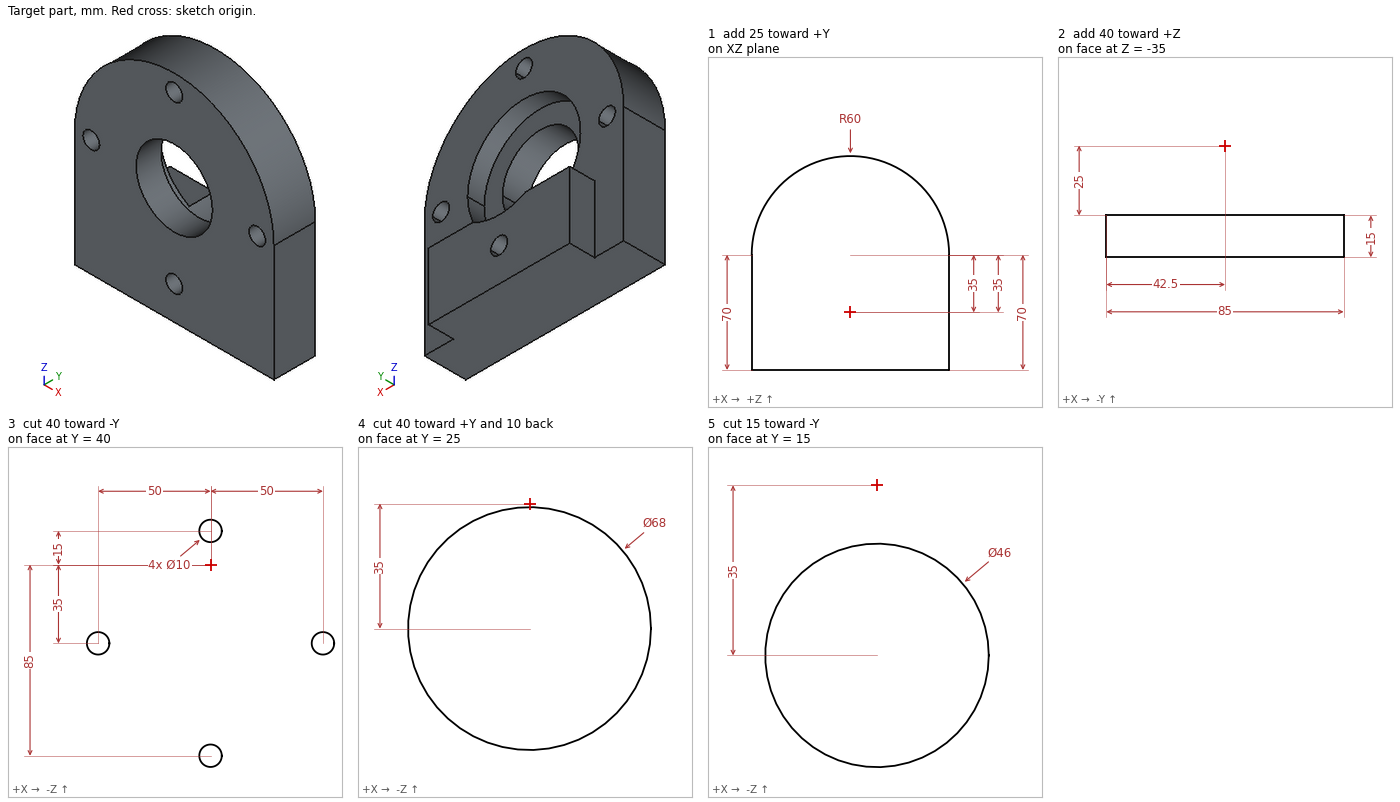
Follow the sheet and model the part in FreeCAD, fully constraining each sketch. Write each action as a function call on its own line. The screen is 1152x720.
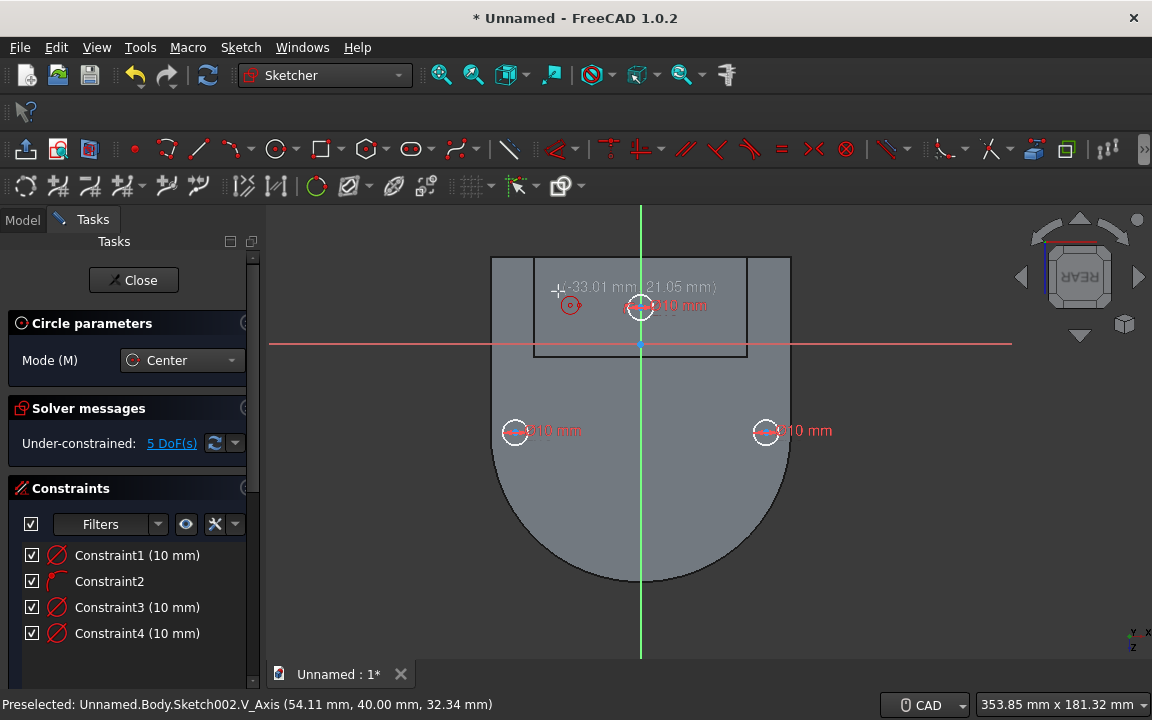
scroll(641, 557, up, 3)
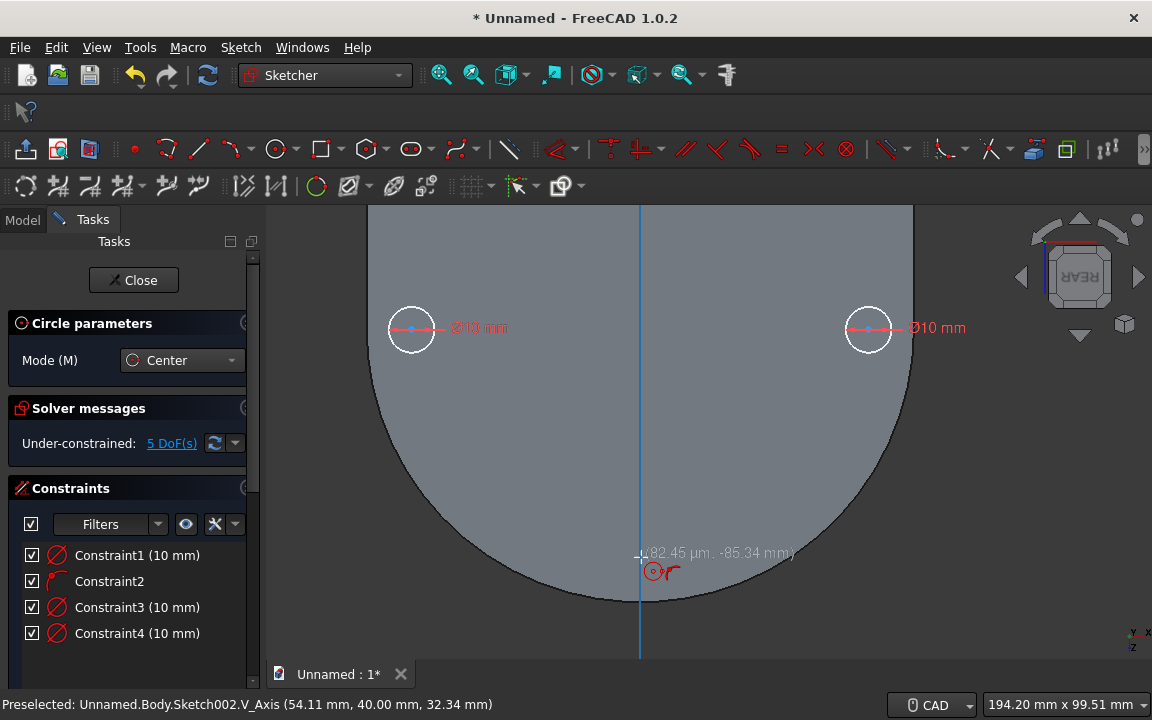
click(640, 557)
move(656, 541)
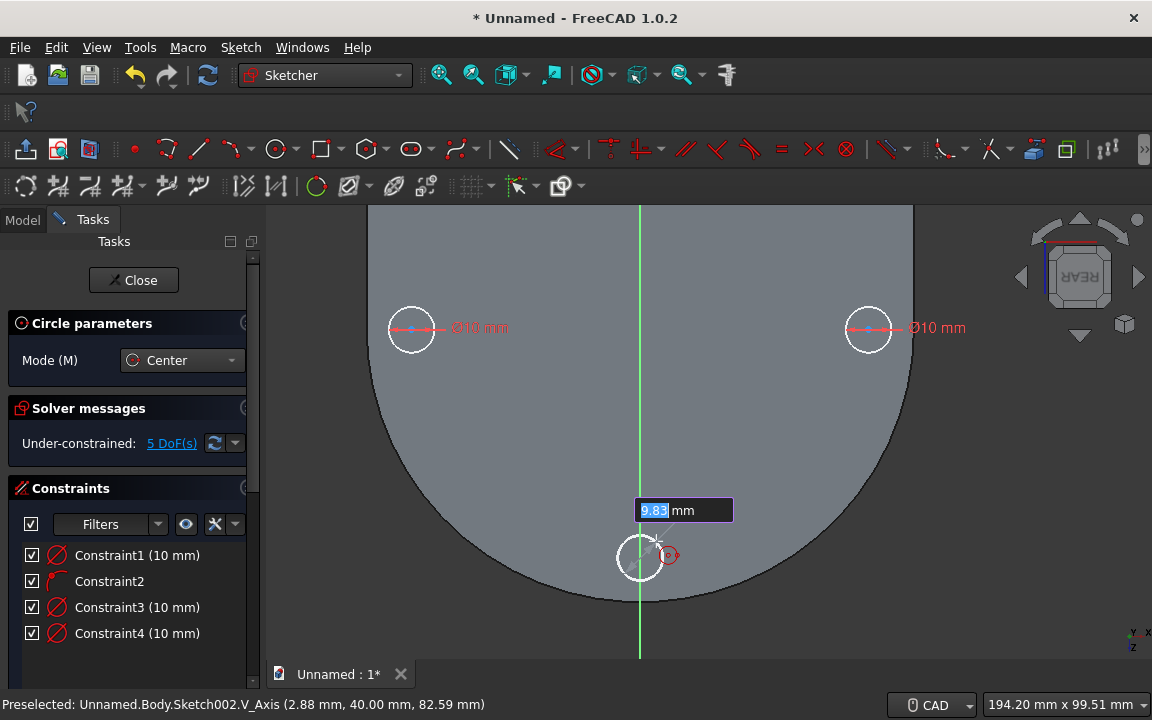
text(10)
key(Return)
key(Escape)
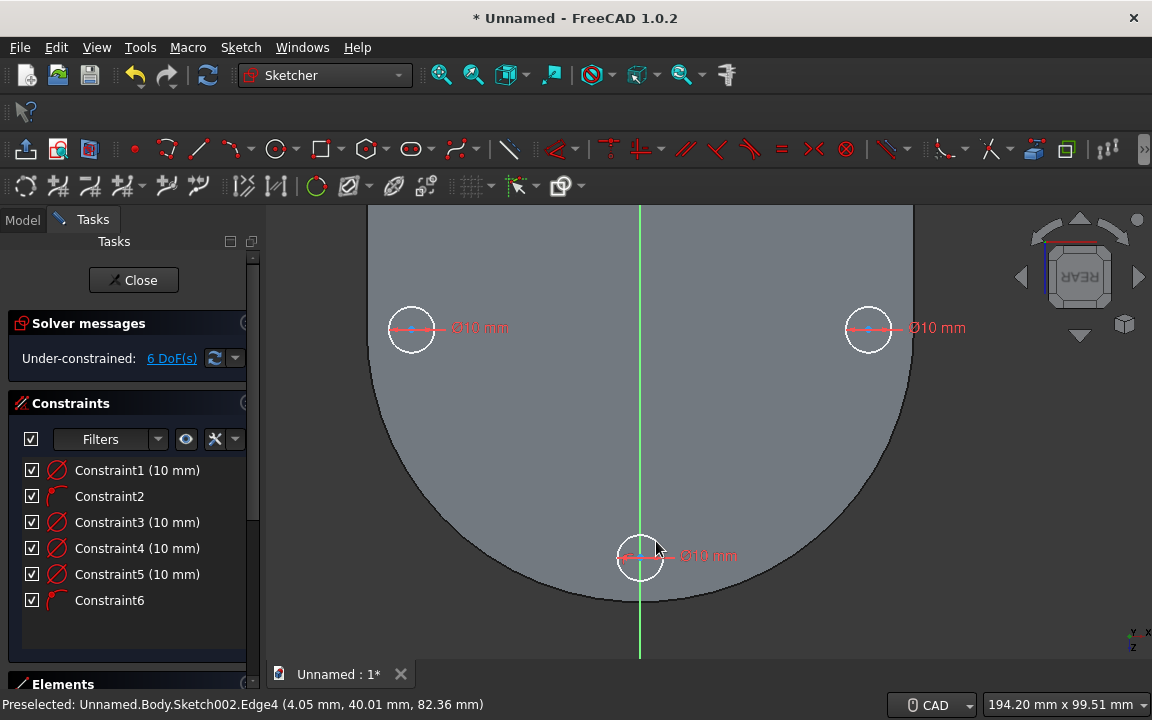
click(412, 330)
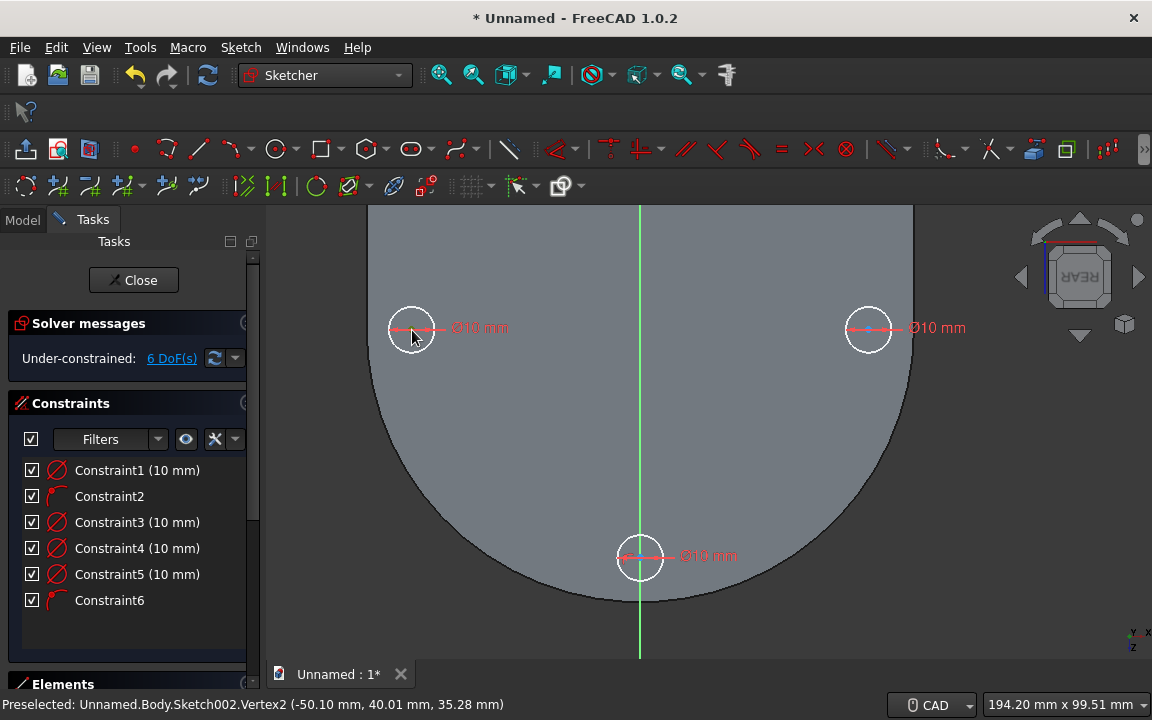
click(869, 330)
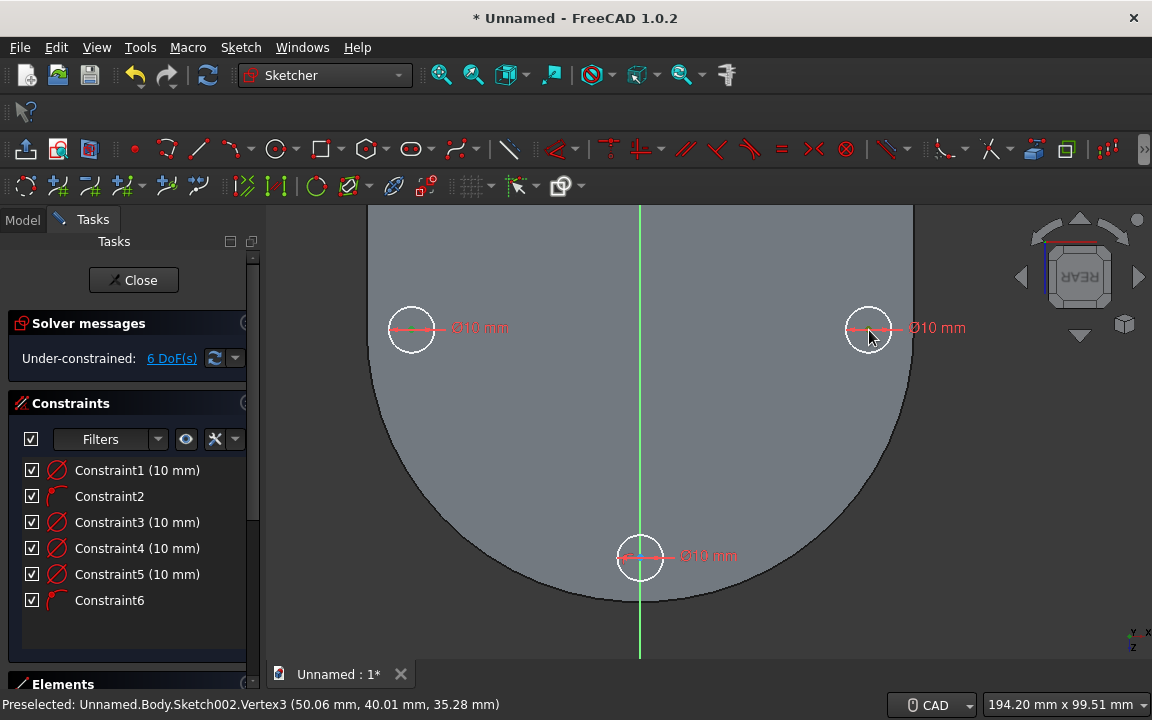
key(h)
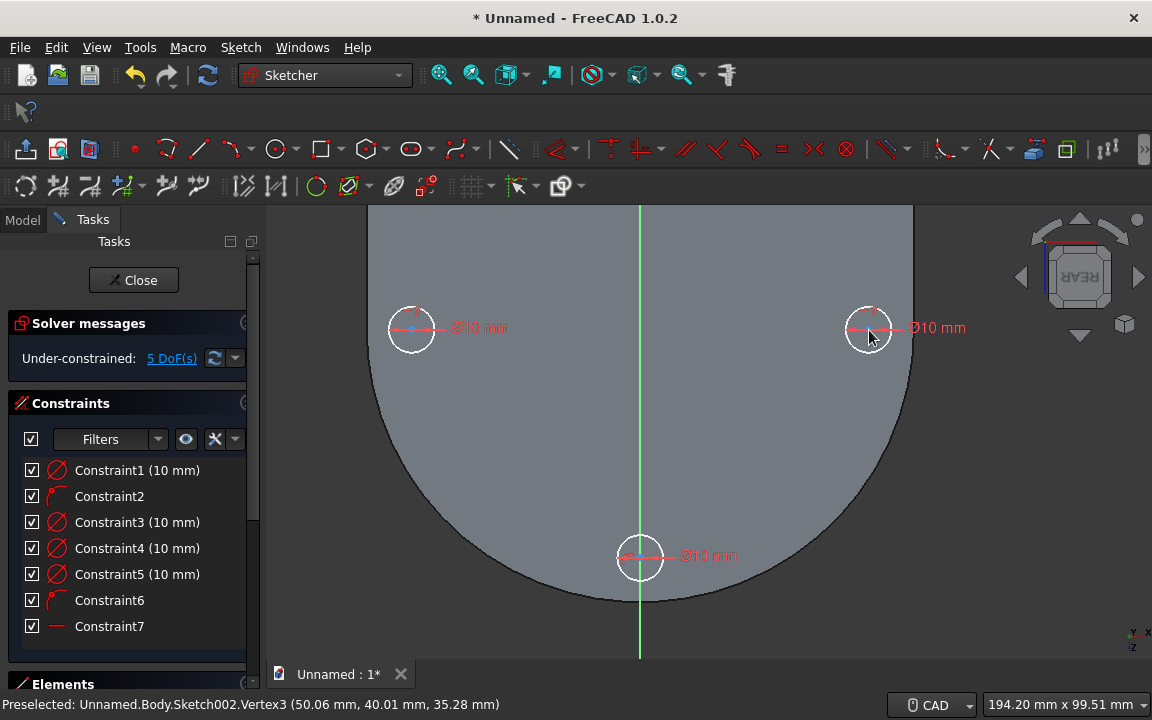
click(556, 150)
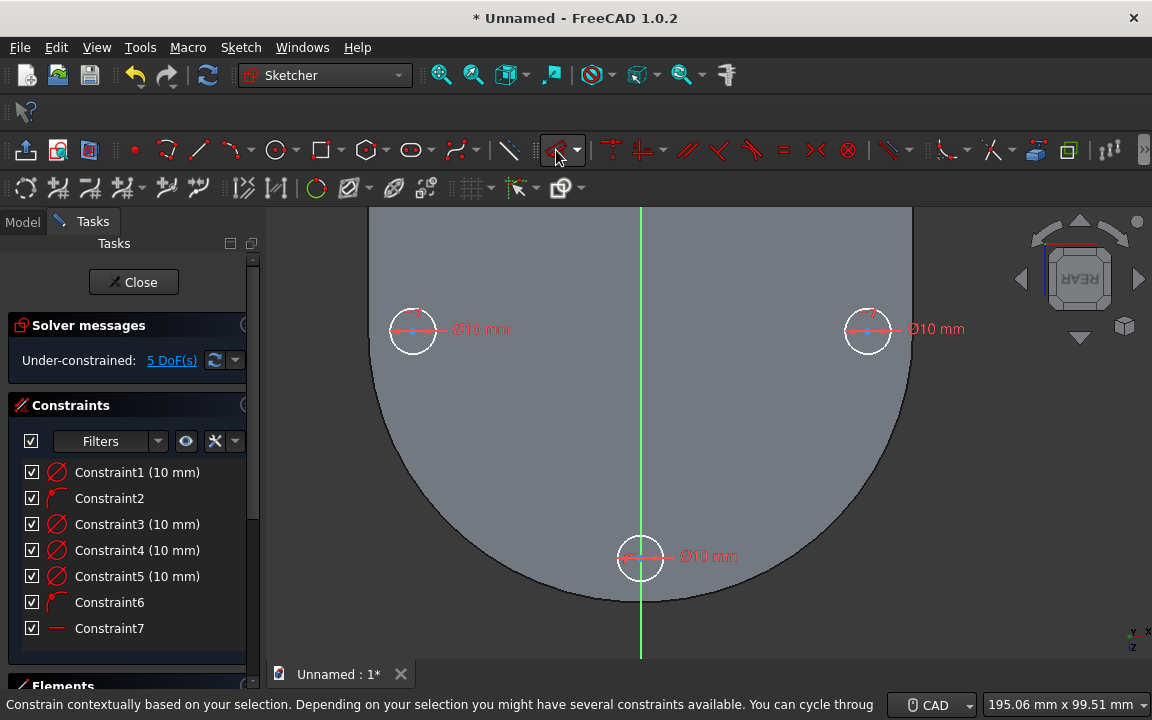
scroll(640, 558, down, 3)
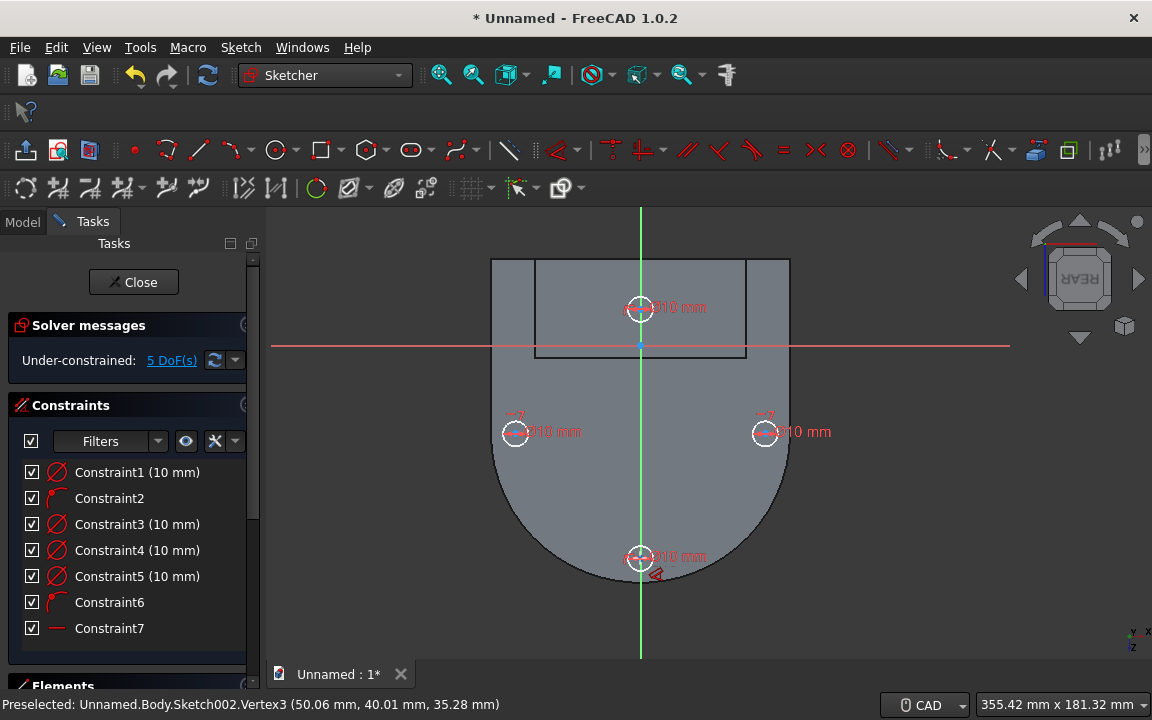
click(641, 309)
click(675, 328)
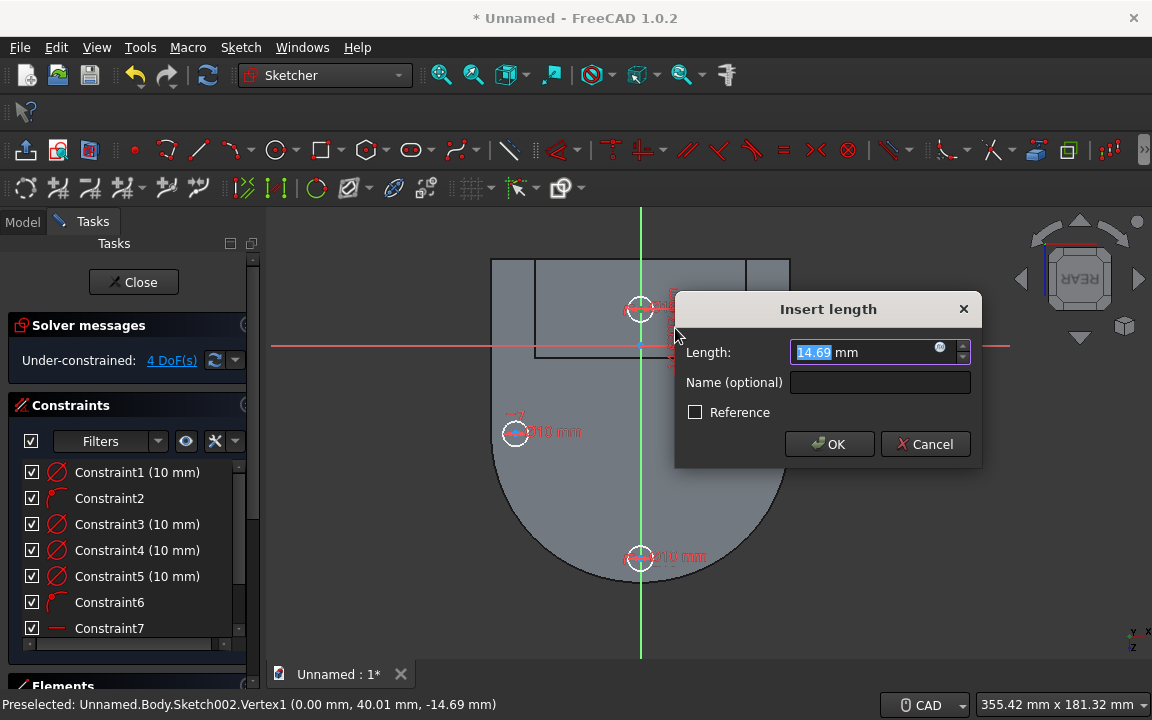
text(15)
key(Return)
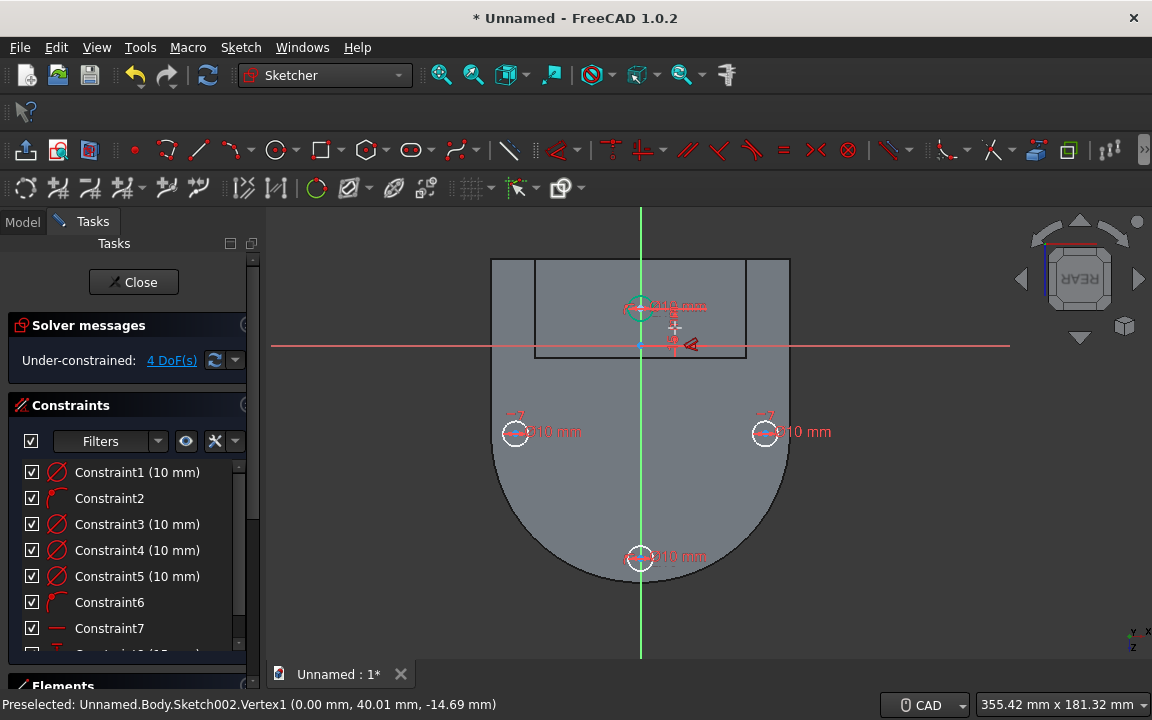
click(516, 434)
click(578, 312)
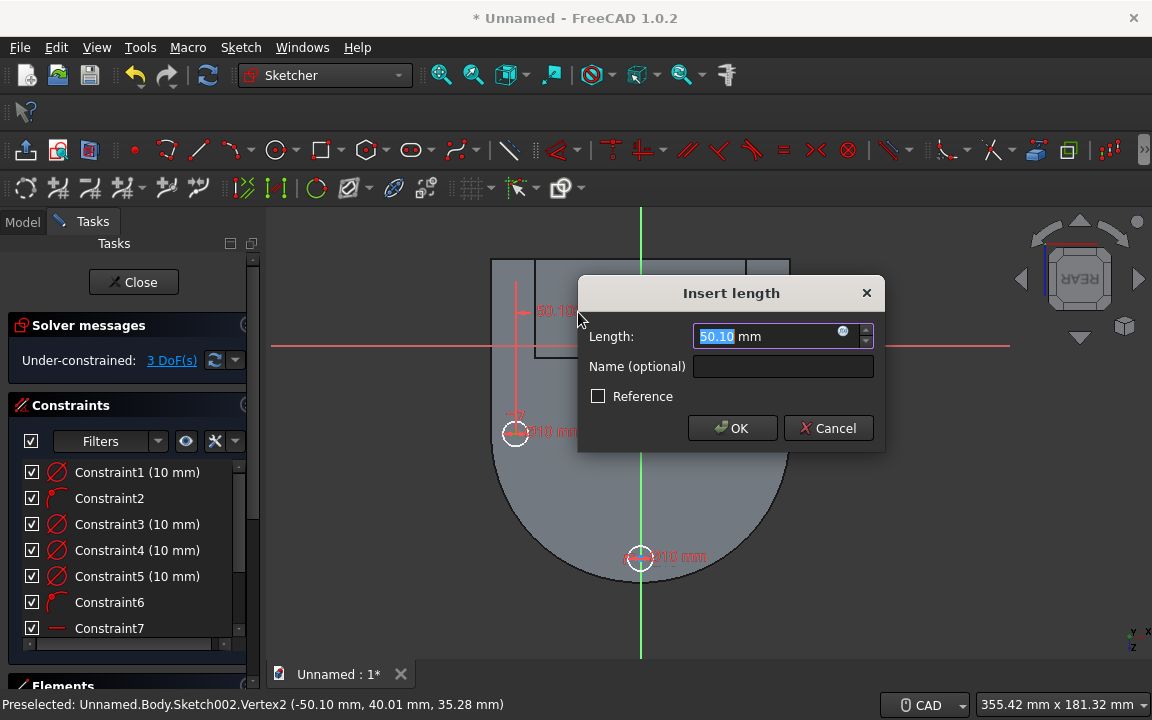
text(50)
key(Return)